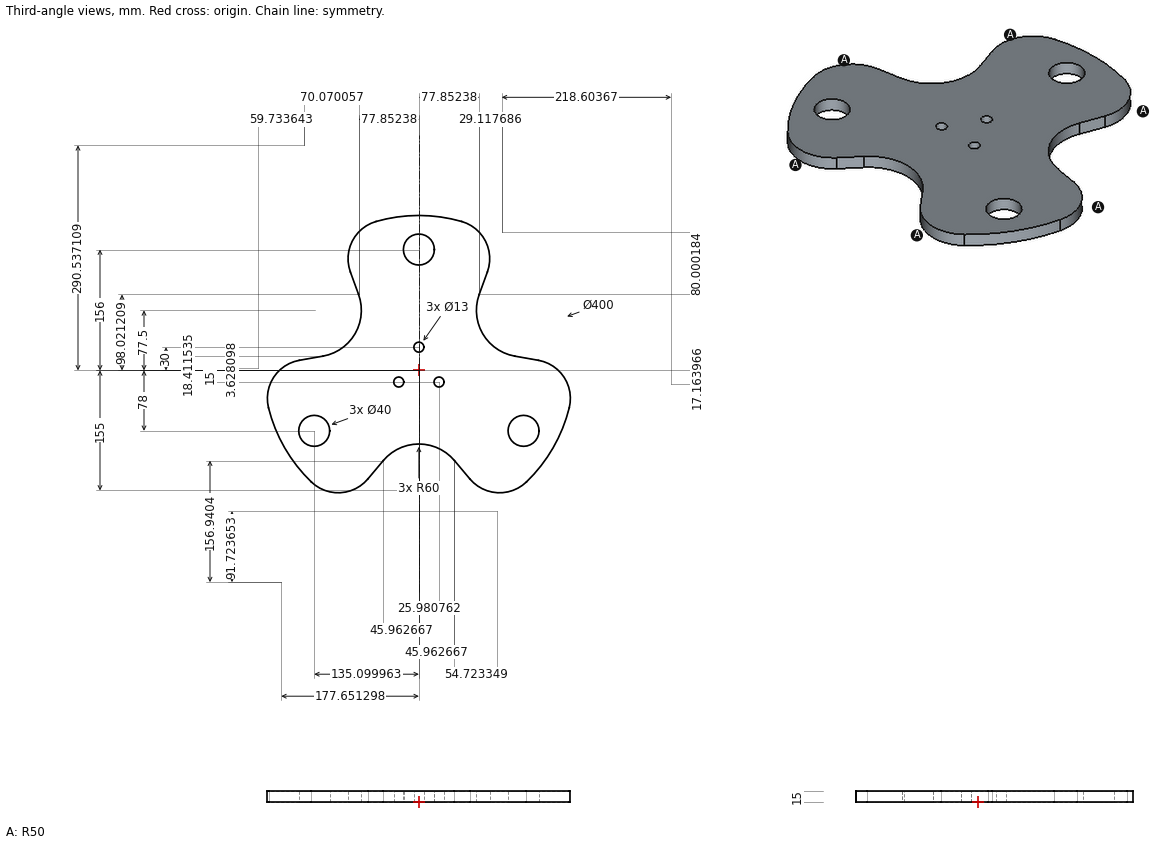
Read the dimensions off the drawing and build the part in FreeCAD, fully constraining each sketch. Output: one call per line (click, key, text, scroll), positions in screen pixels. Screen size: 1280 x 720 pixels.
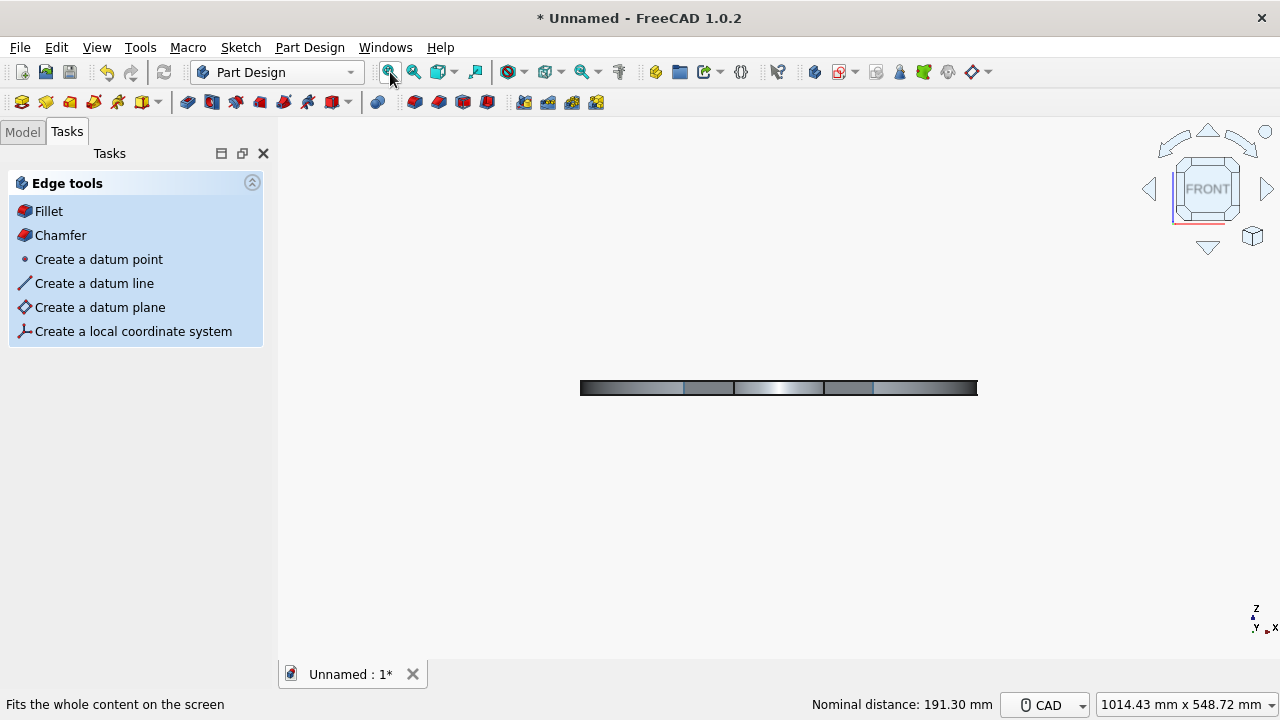
click(390, 72)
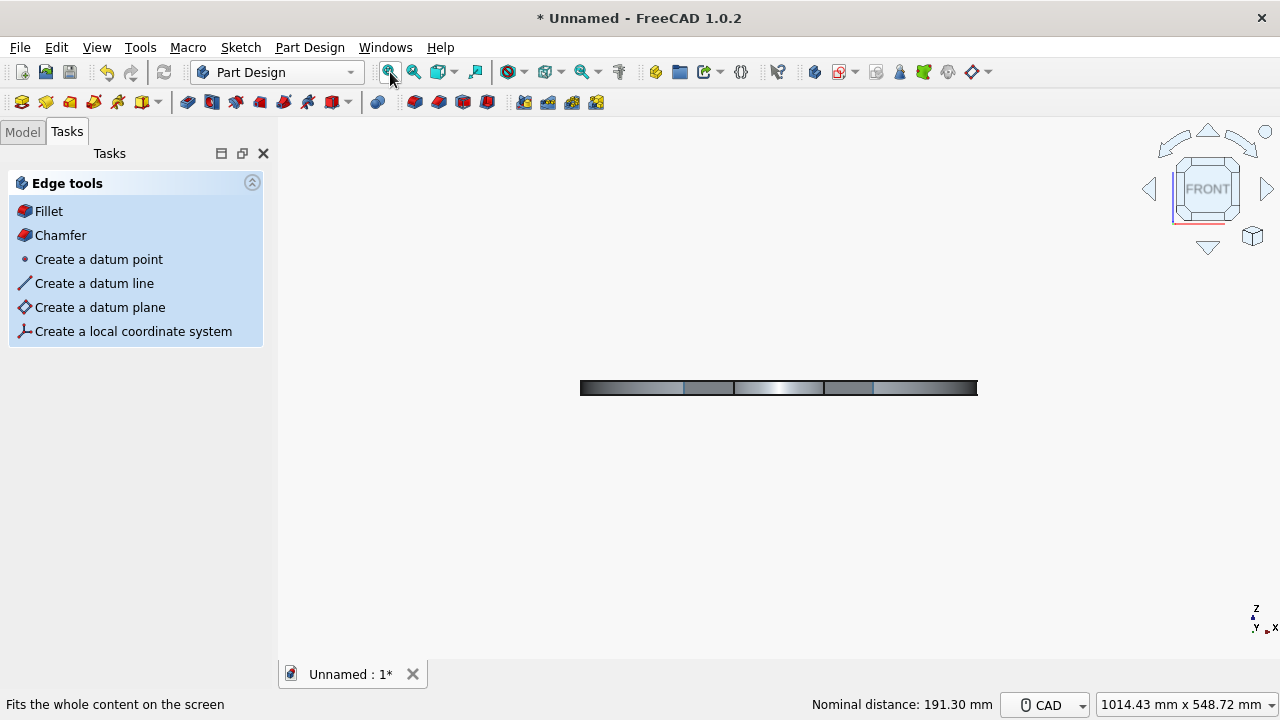
scroll(976, 387, up, 5)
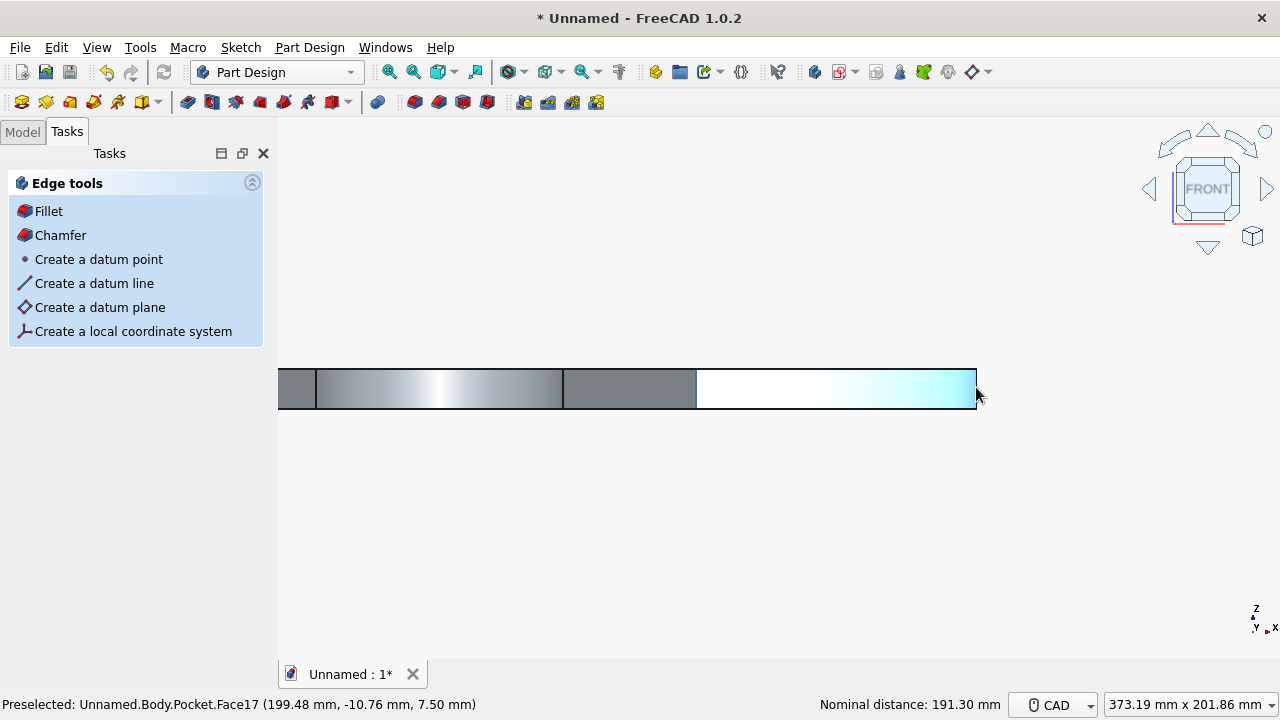
click(390, 72)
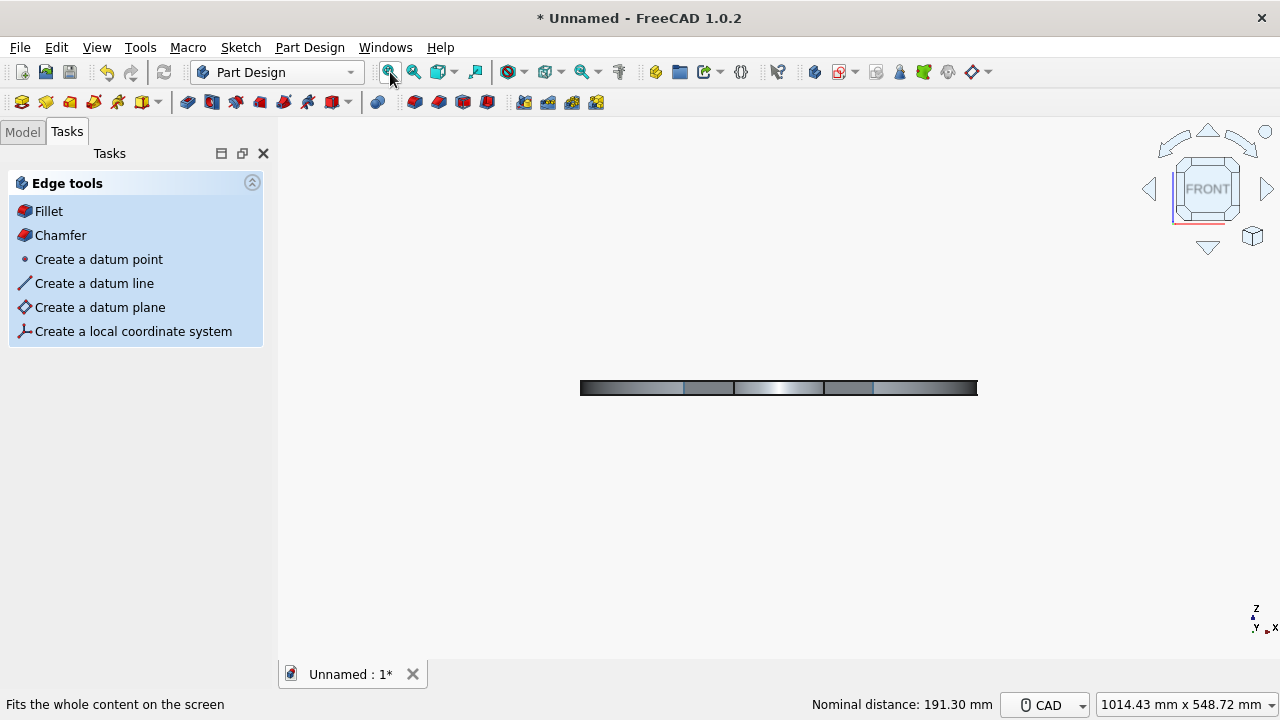
key(3)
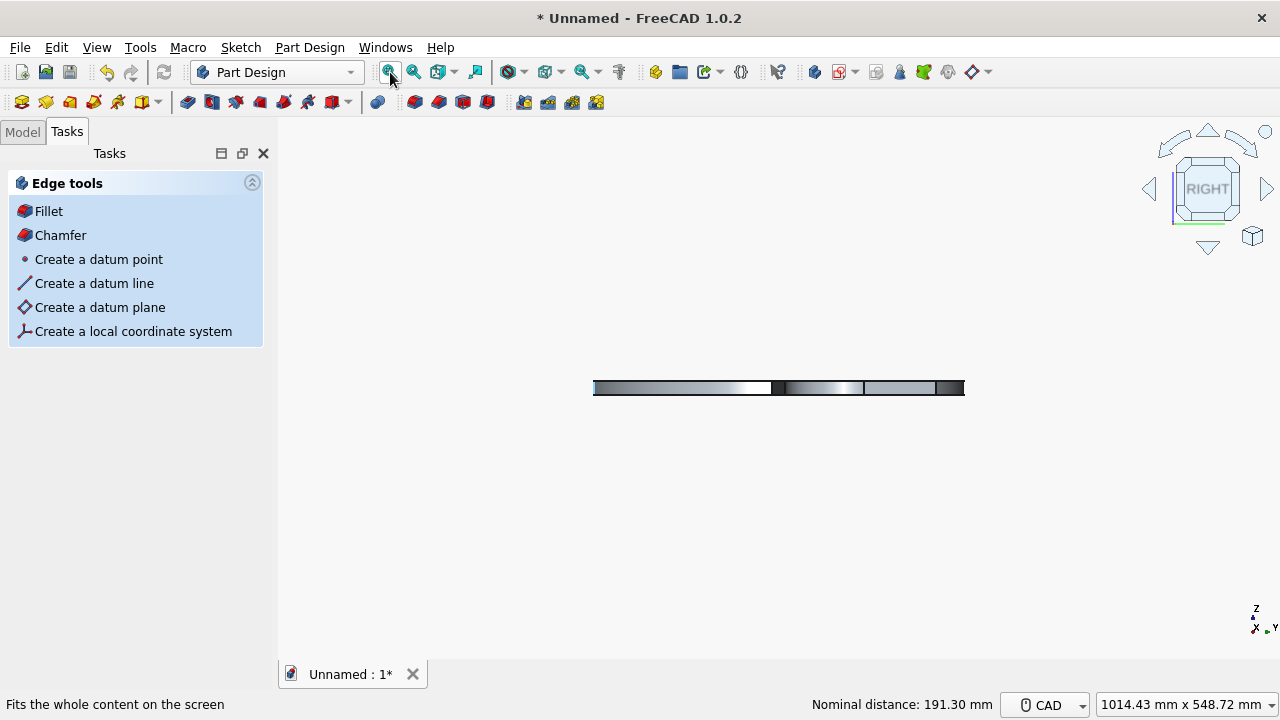
click(390, 72)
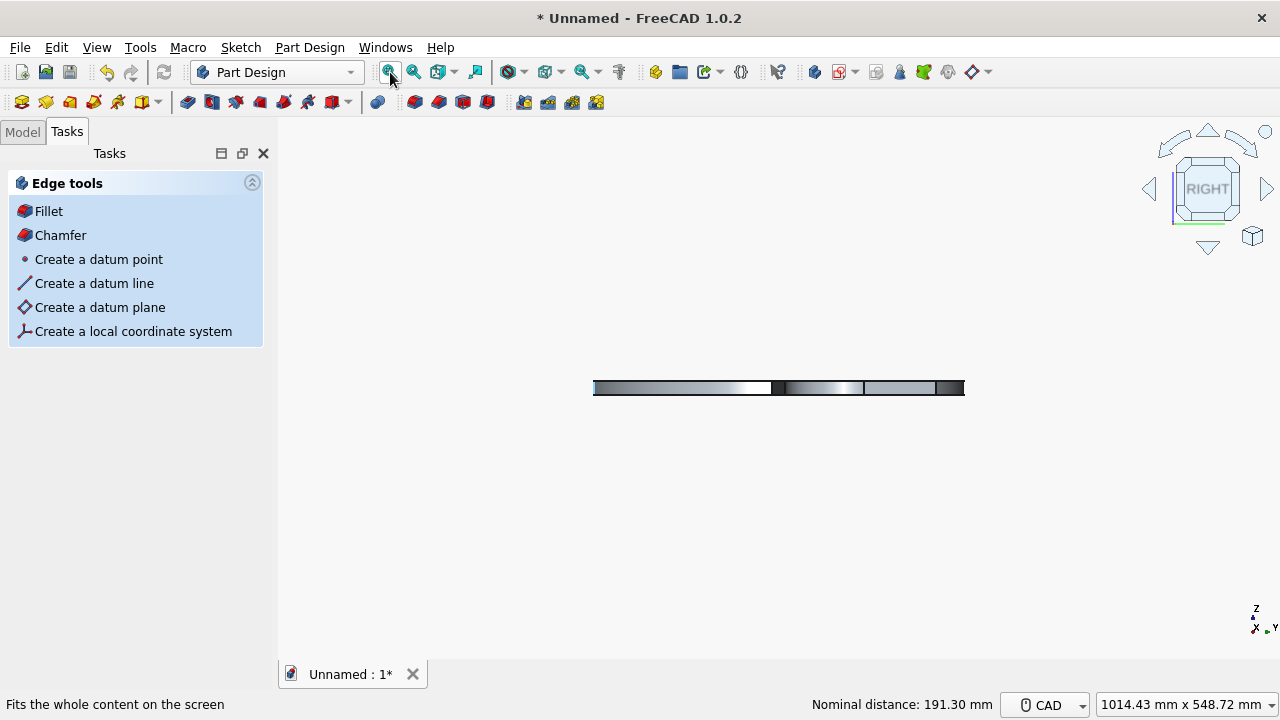
click(936, 387, ctrl)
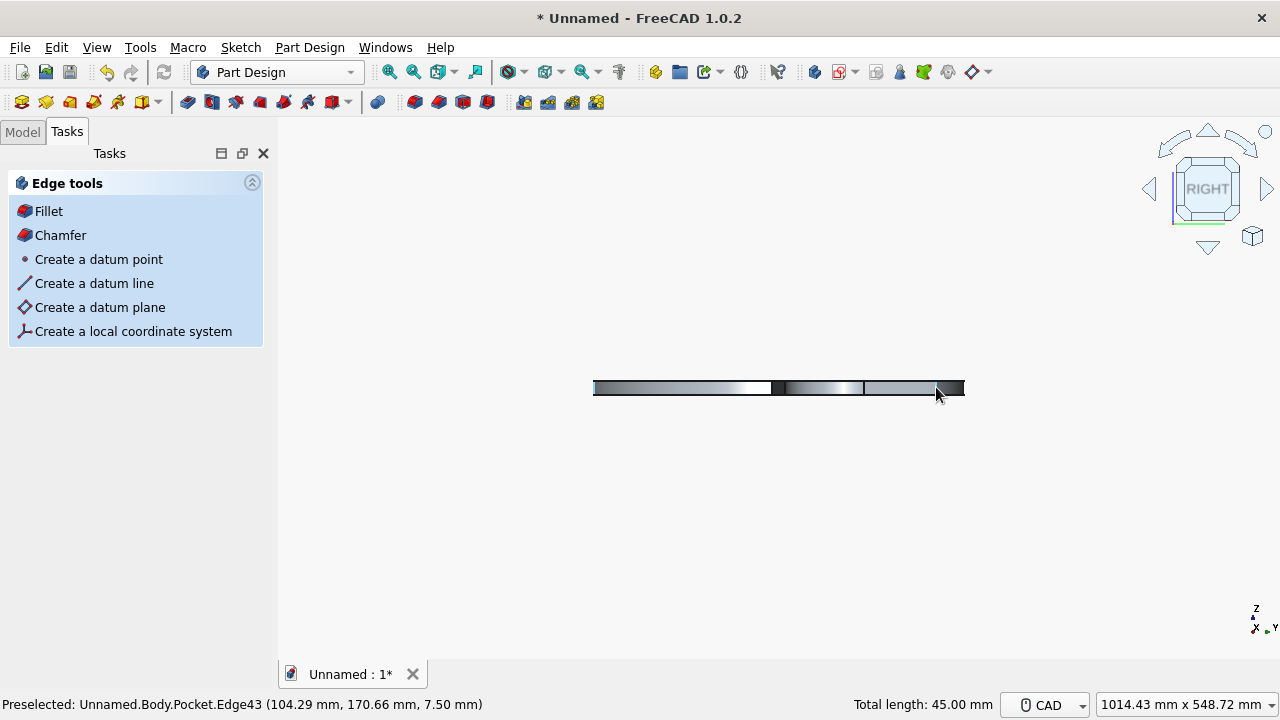
scroll(772, 387, up, 5)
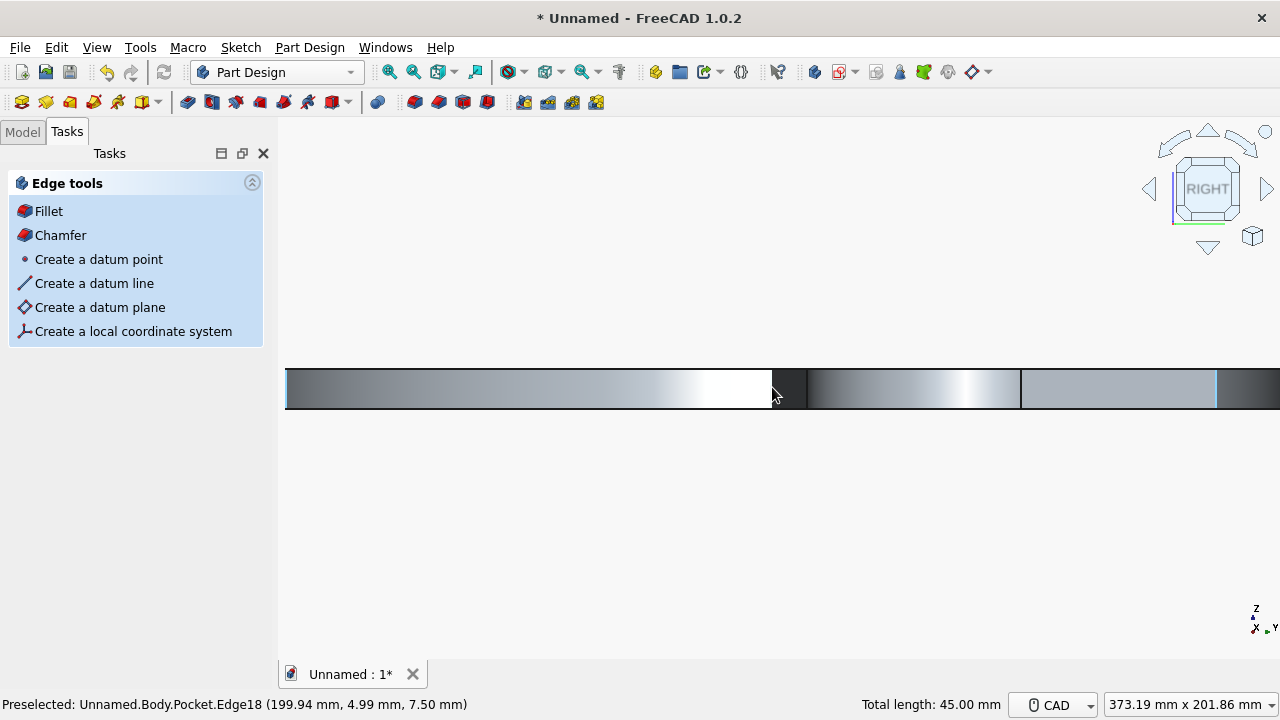
click(390, 72)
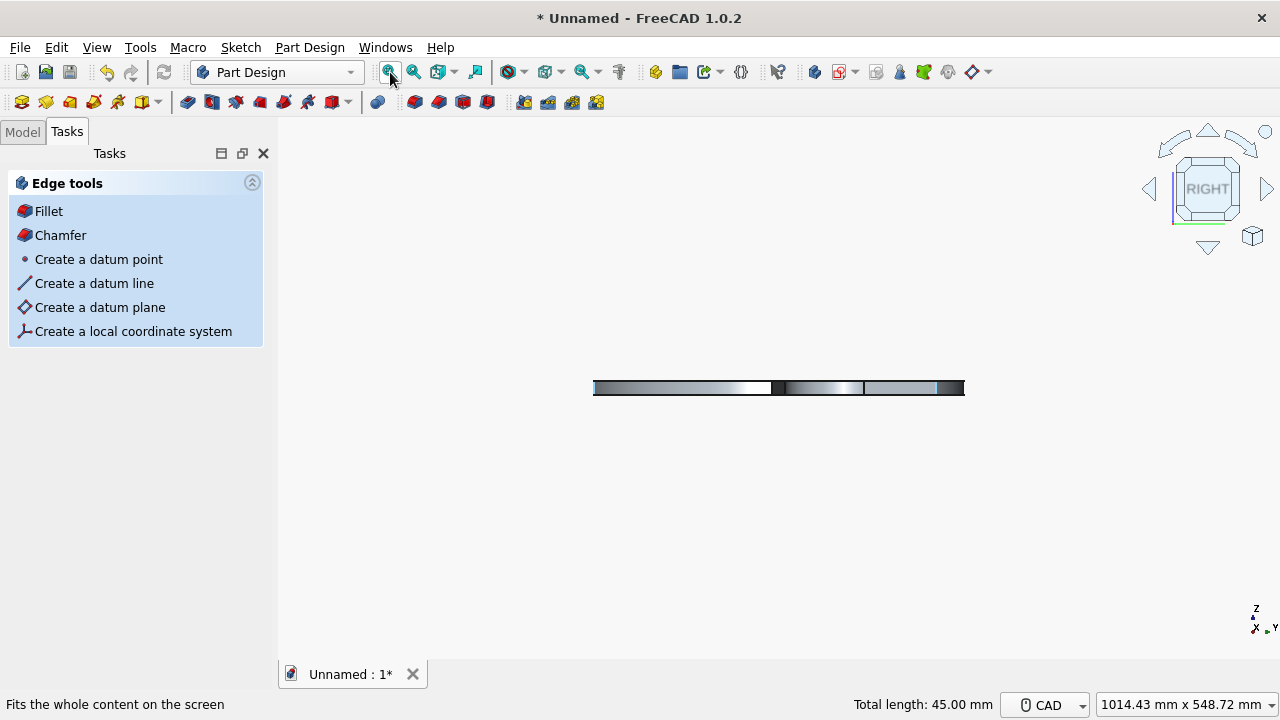
key(5)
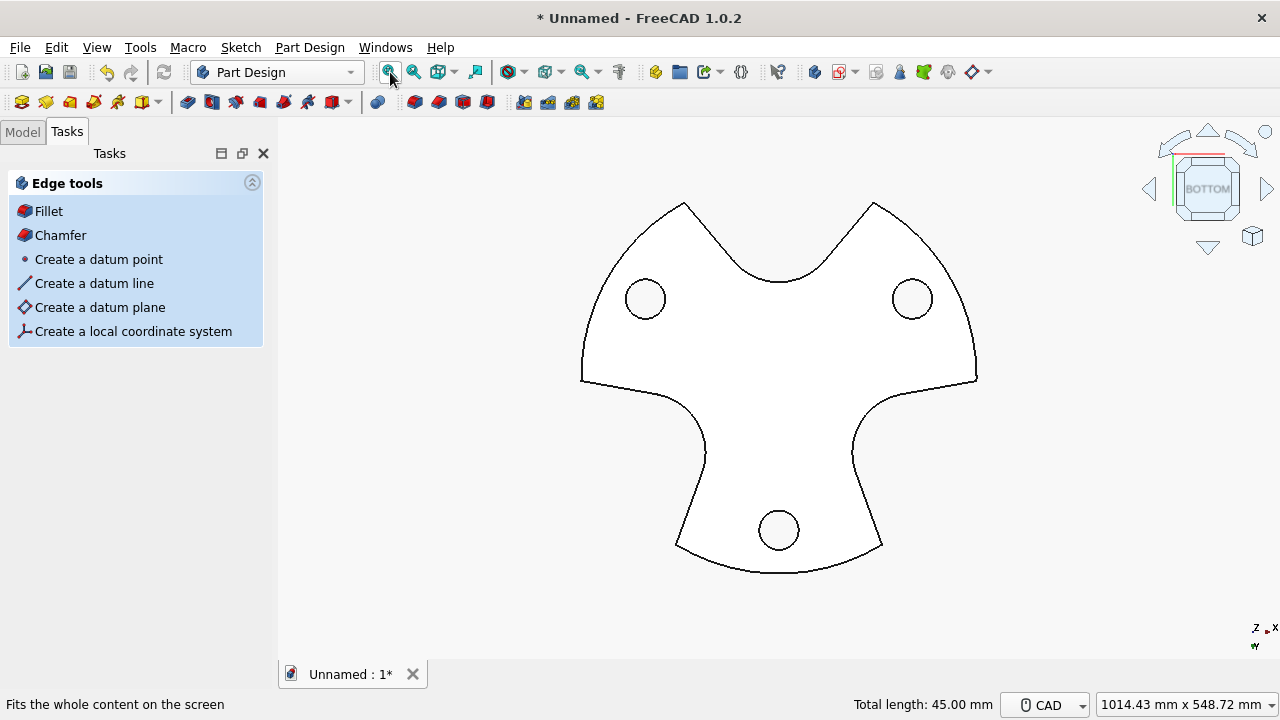
scroll(976, 380, up, 5)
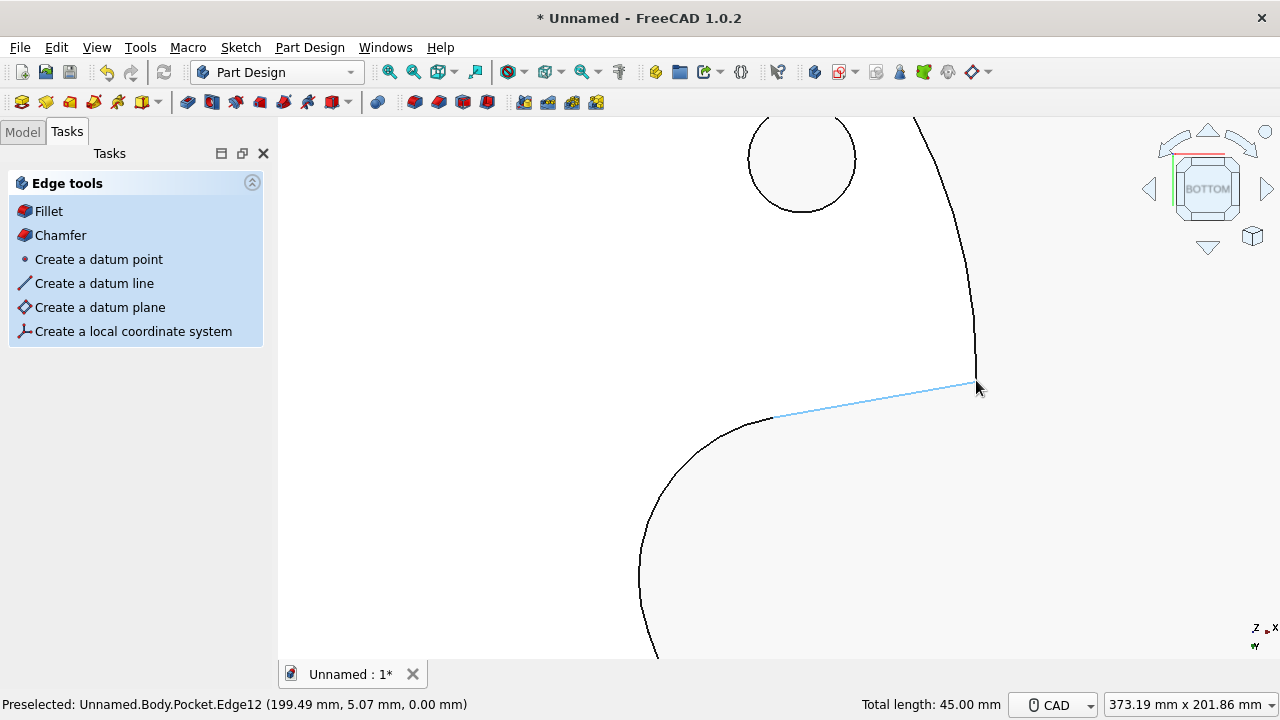
click(390, 72)